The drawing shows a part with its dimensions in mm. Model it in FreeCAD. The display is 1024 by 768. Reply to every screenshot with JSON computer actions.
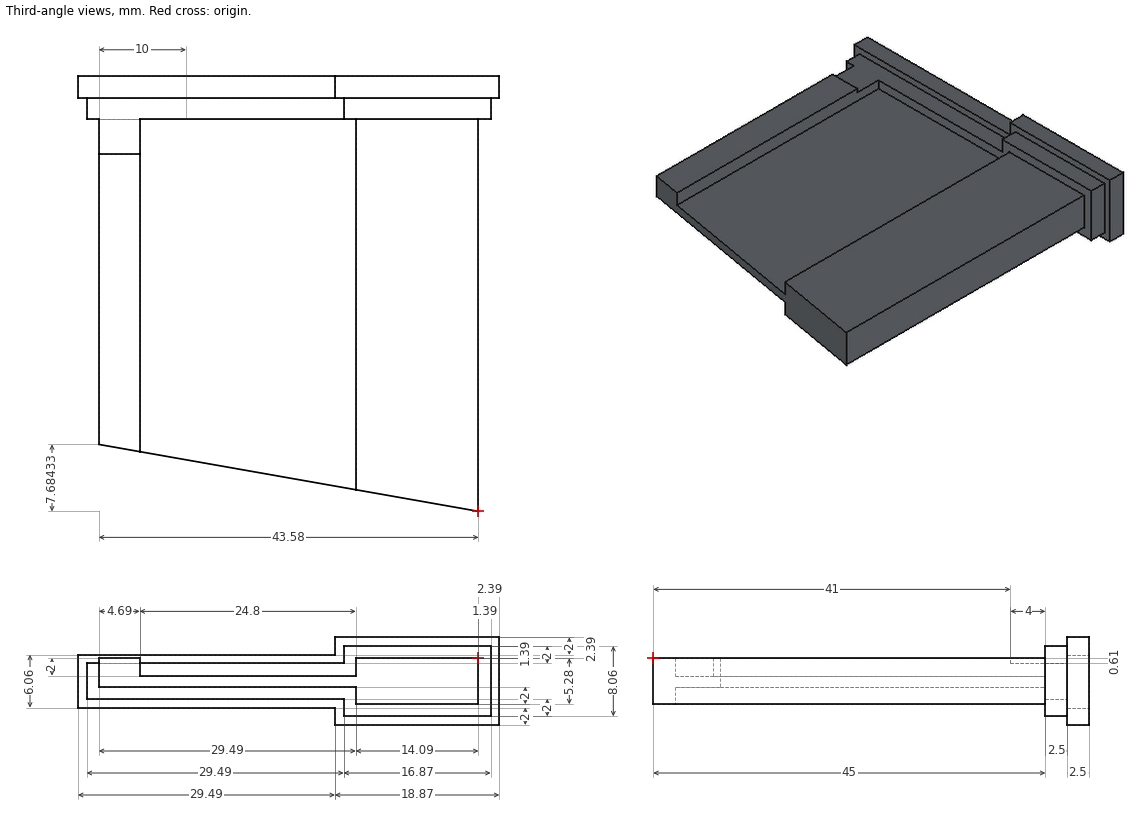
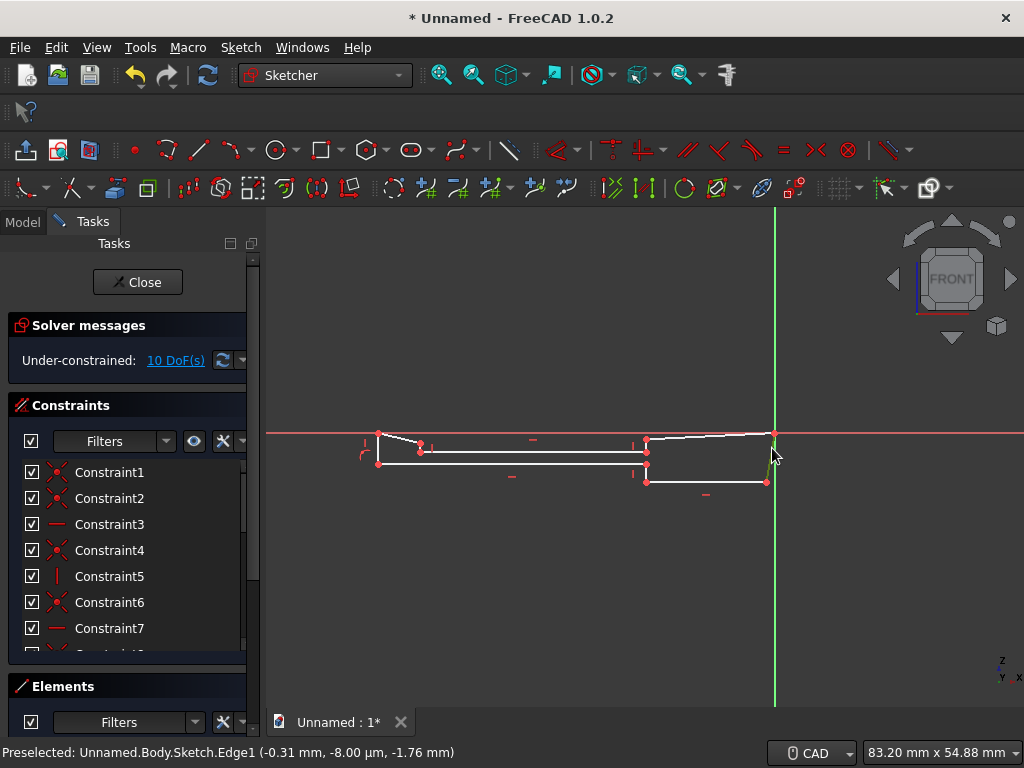
{"action": "left_click", "coordinate": [666, 150]}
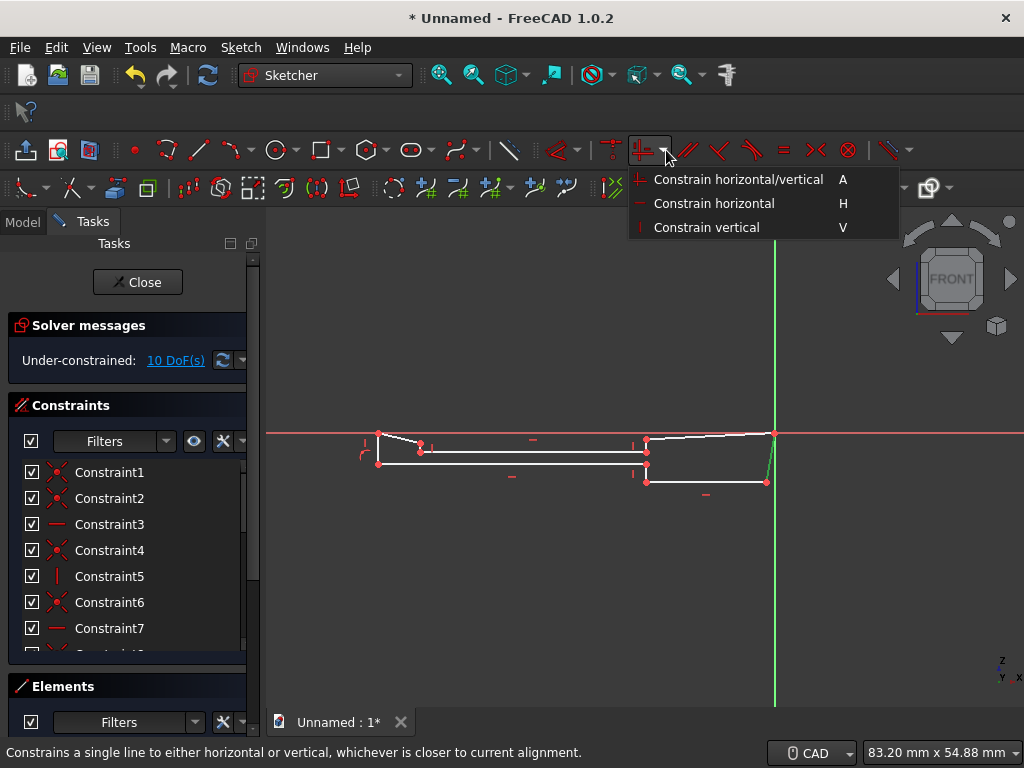
{"action": "left_click", "coordinate": [764, 227]}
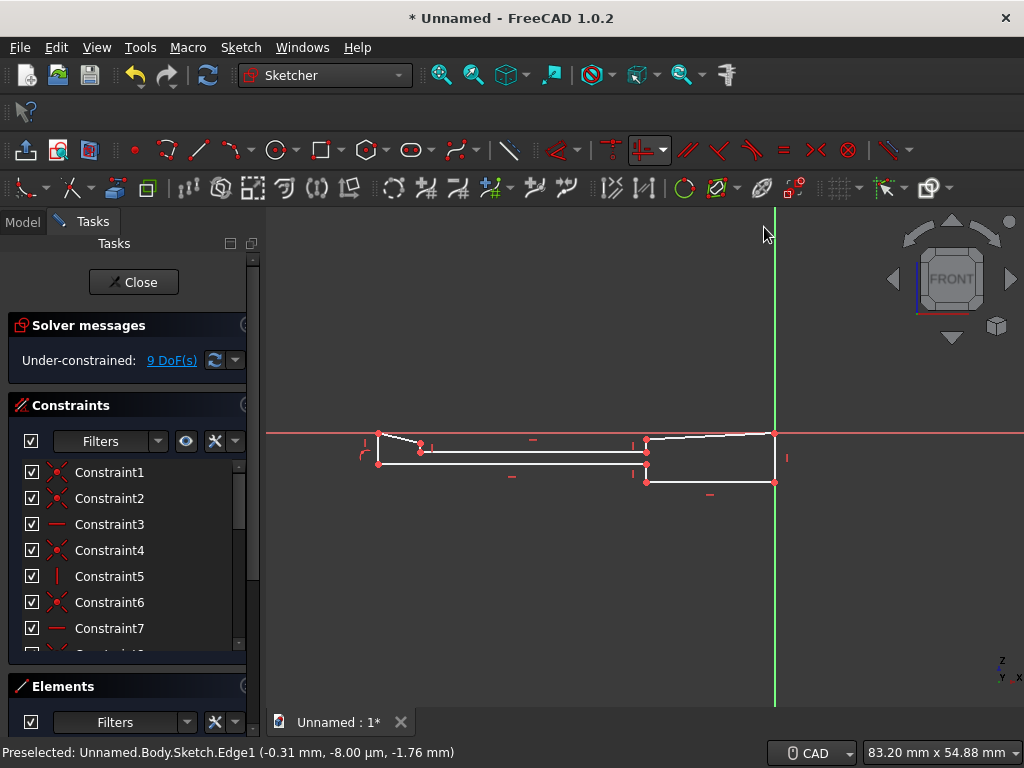
{"action": "left_click", "coordinate": [391, 436]}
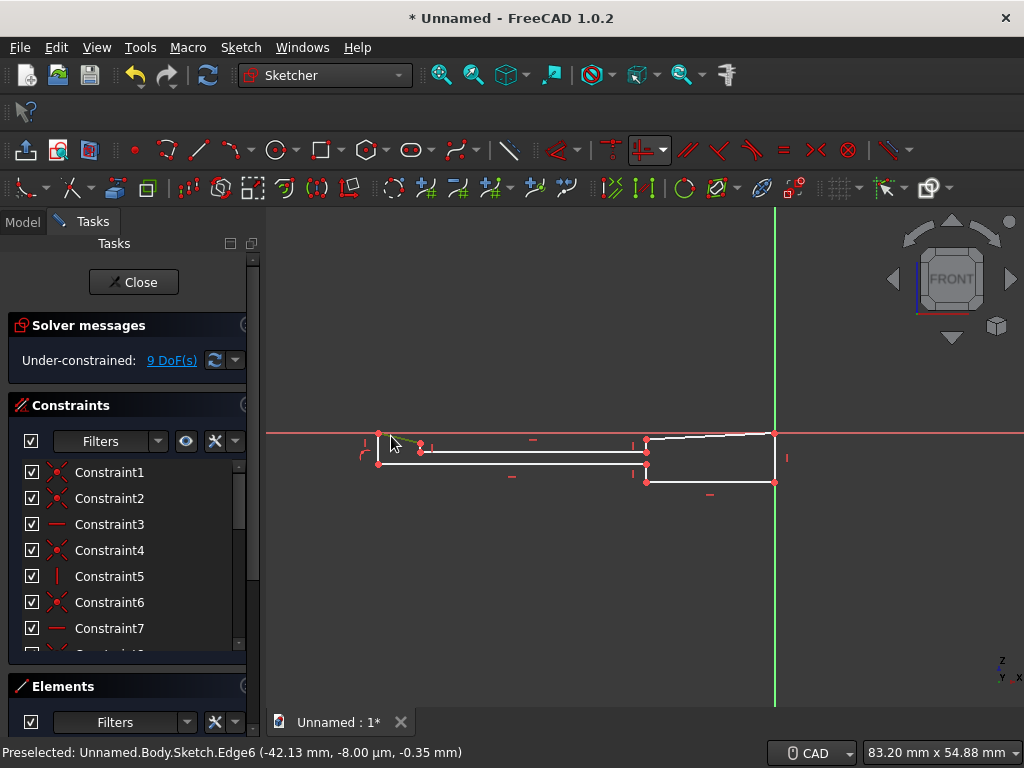
{"action": "key", "text": "h"}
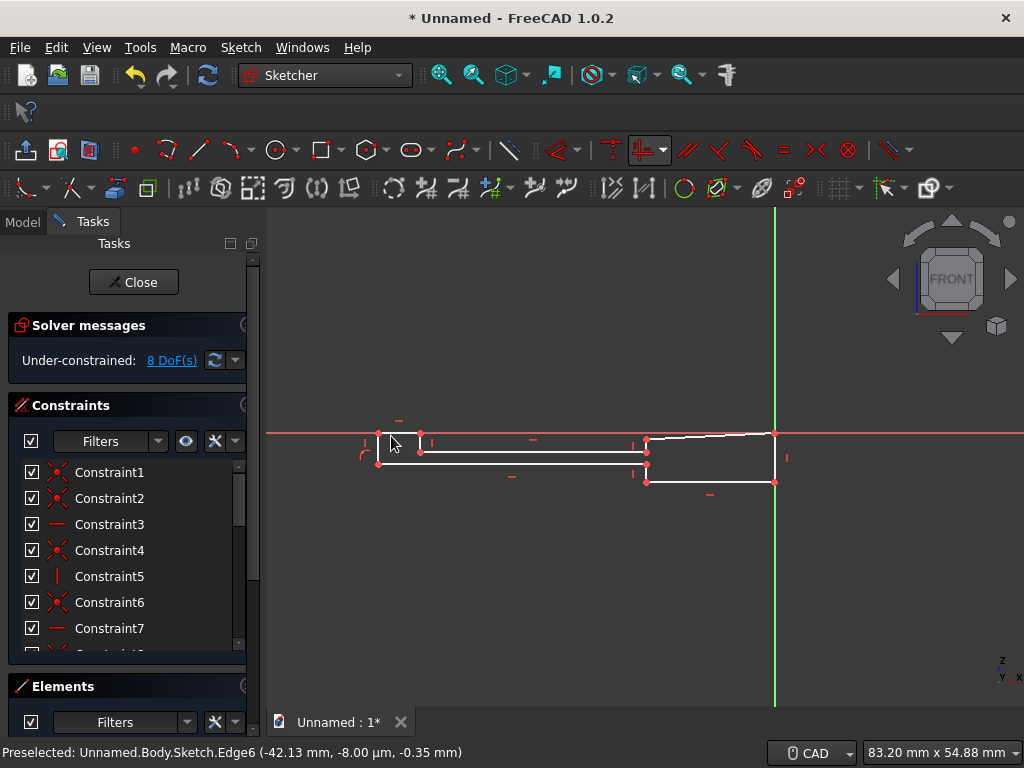
{"action": "left_click", "coordinate": [736, 435]}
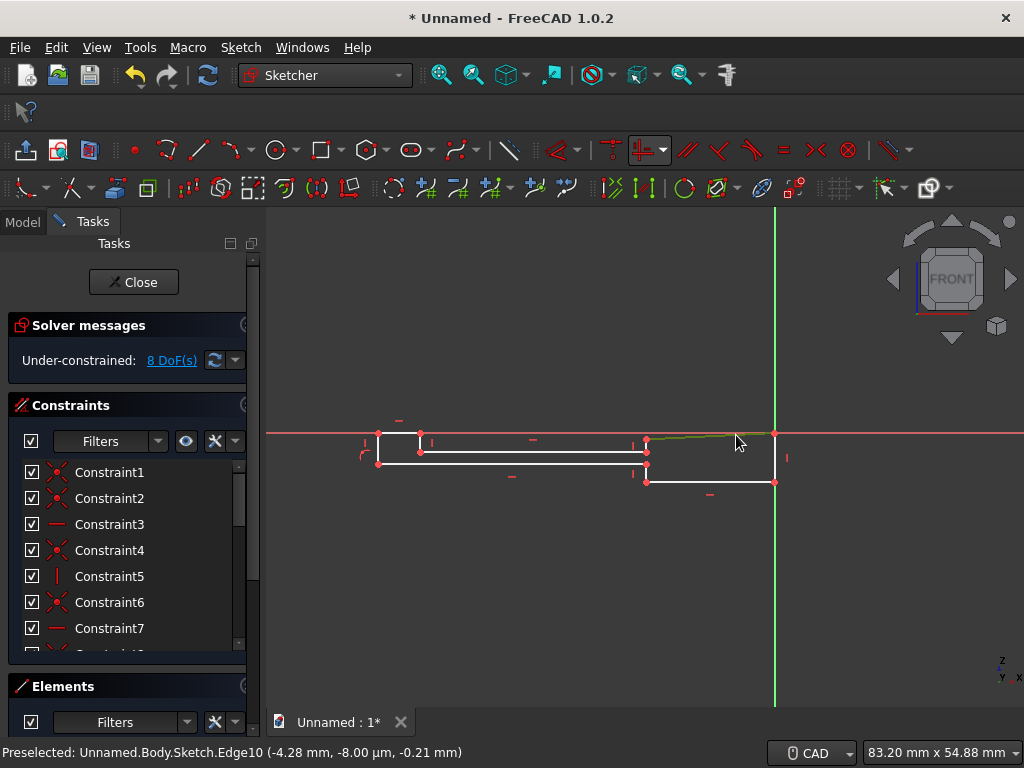
{"action": "key", "text": "h"}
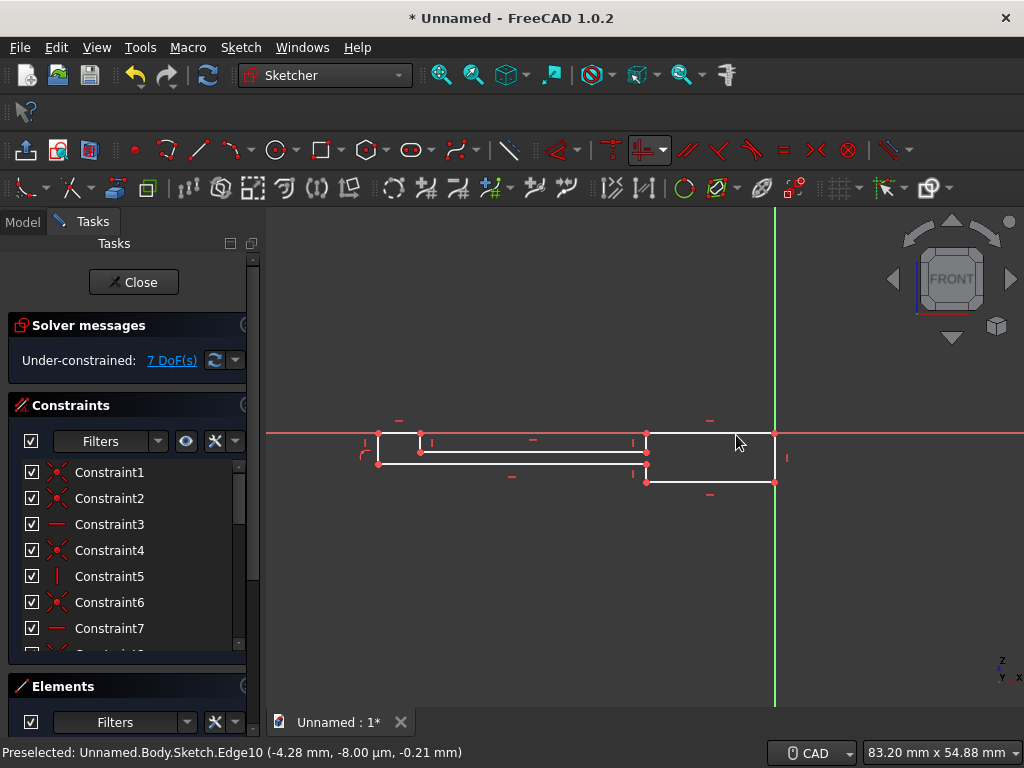
{"action": "key", "text": "d"}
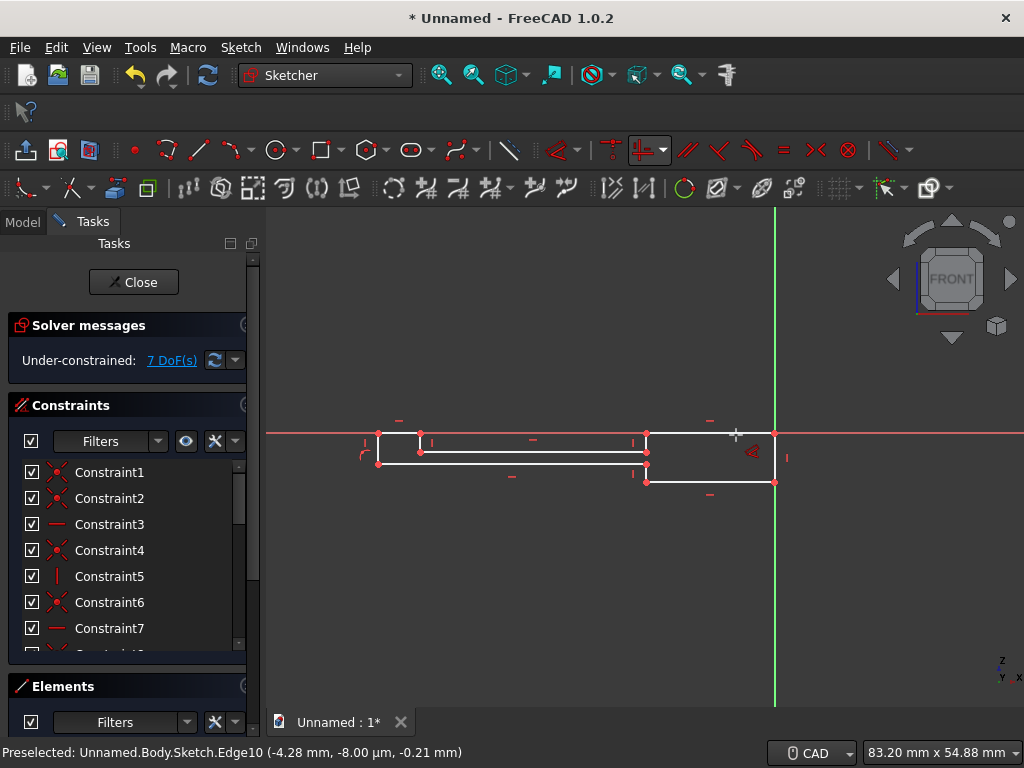
{"action": "scroll", "coordinate": [646, 473], "scroll_direction": "up", "scroll_amount": 4}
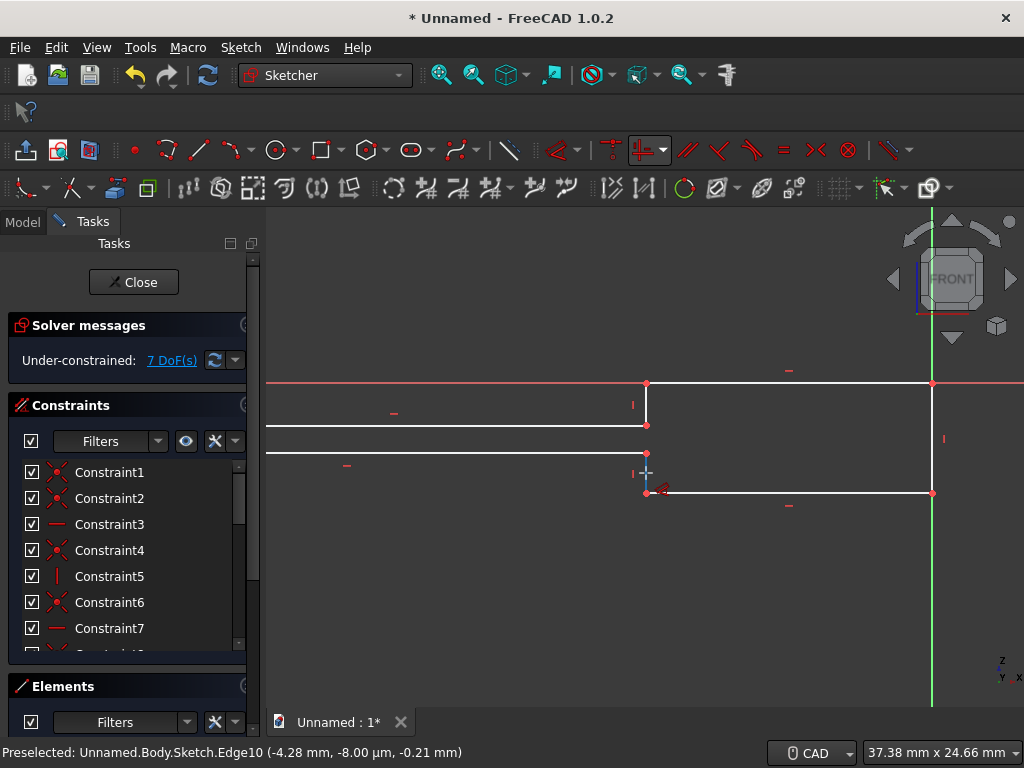
{"action": "left_click", "coordinate": [646, 473]}
{"action": "left_click", "coordinate": [680, 473]}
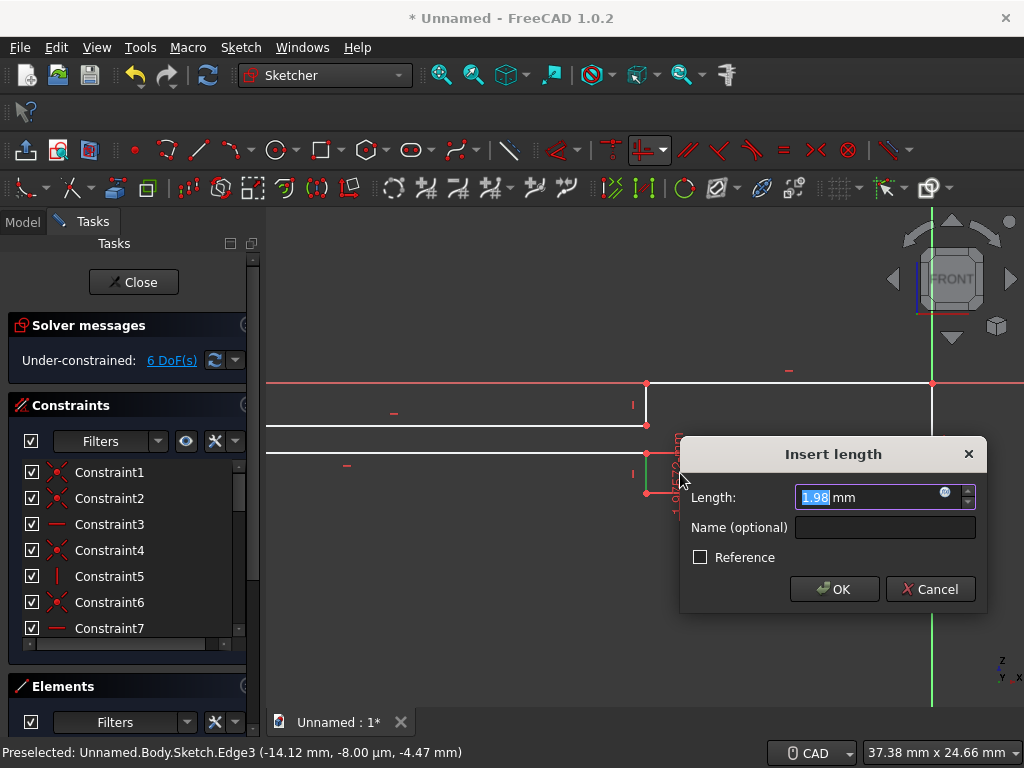
{"action": "type", "text": "2"}
{"action": "key", "text": "Return"}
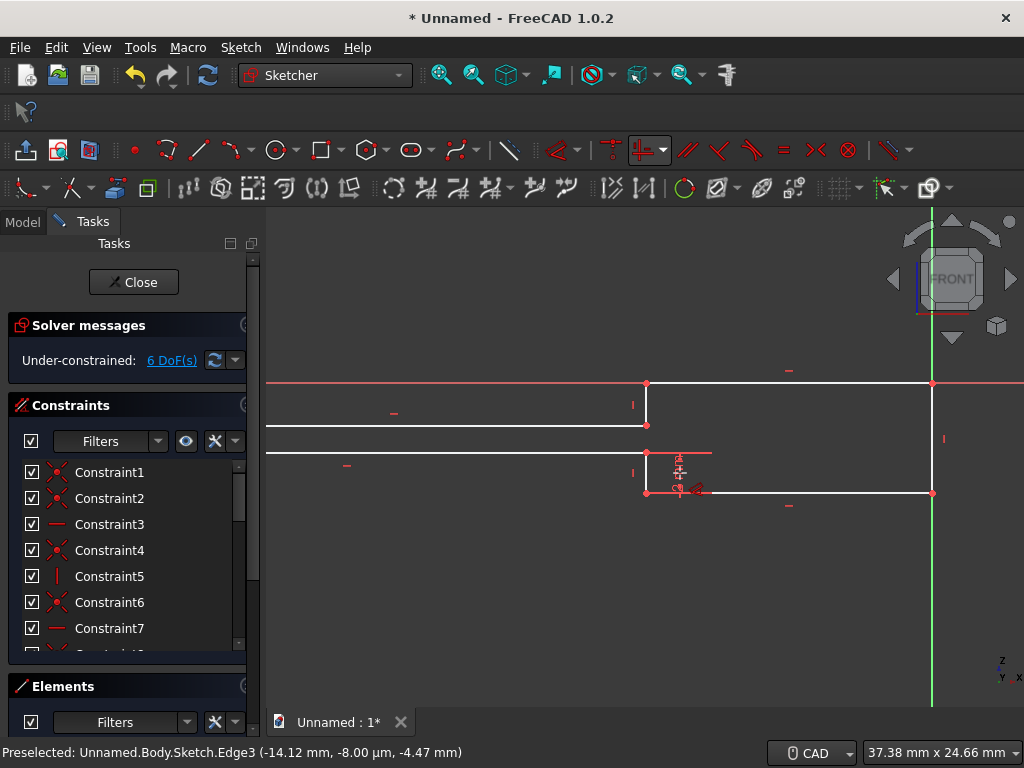
{"action": "scroll", "coordinate": [647, 473], "scroll_direction": "down", "scroll_amount": 4}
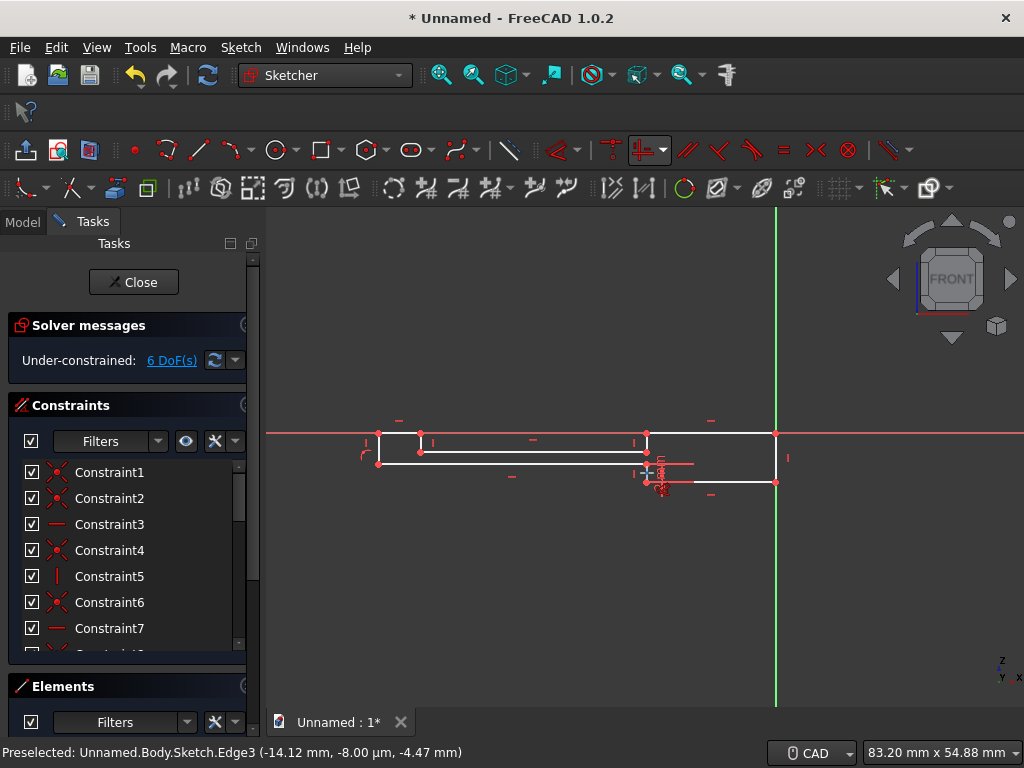
{"action": "scroll", "coordinate": [421, 439], "scroll_direction": "up", "scroll_amount": 5}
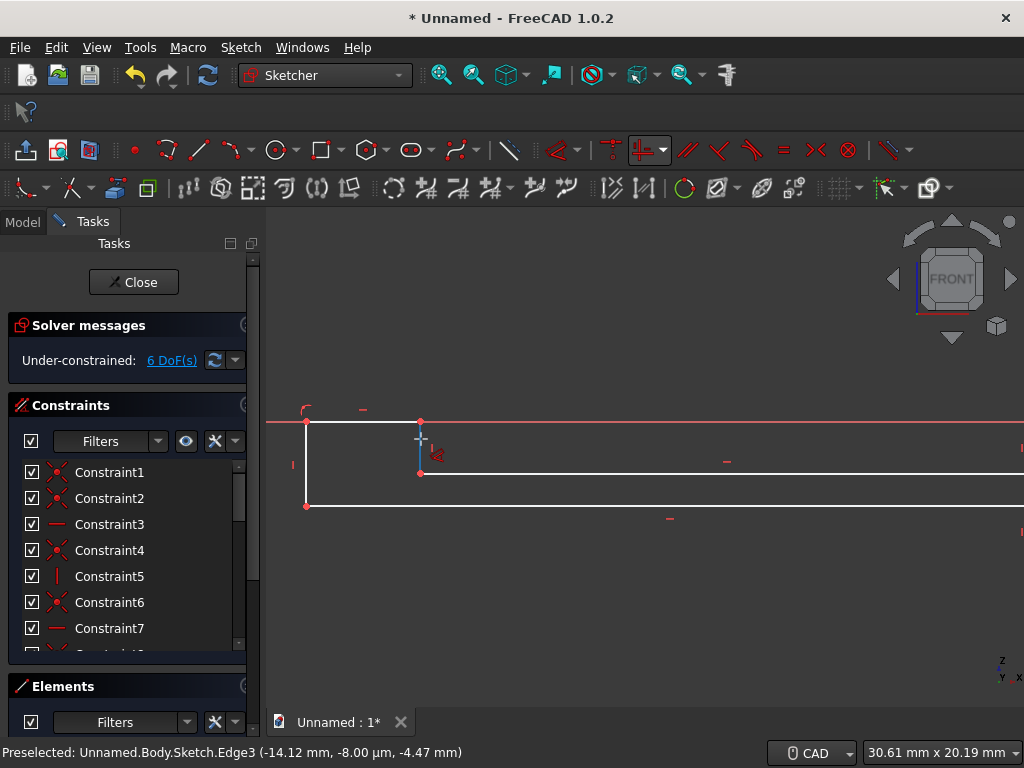
{"action": "left_click", "coordinate": [420, 438]}
{"action": "left_click", "coordinate": [386, 448]}